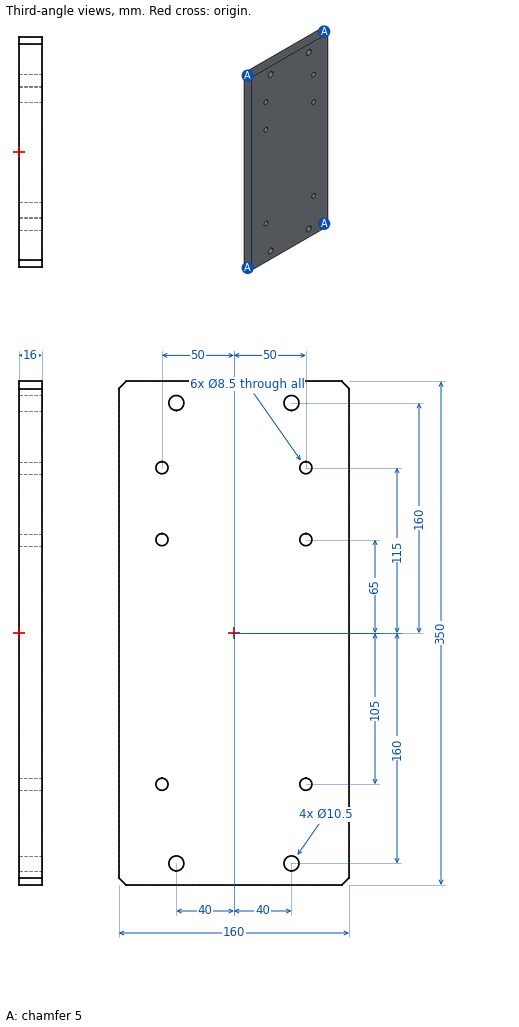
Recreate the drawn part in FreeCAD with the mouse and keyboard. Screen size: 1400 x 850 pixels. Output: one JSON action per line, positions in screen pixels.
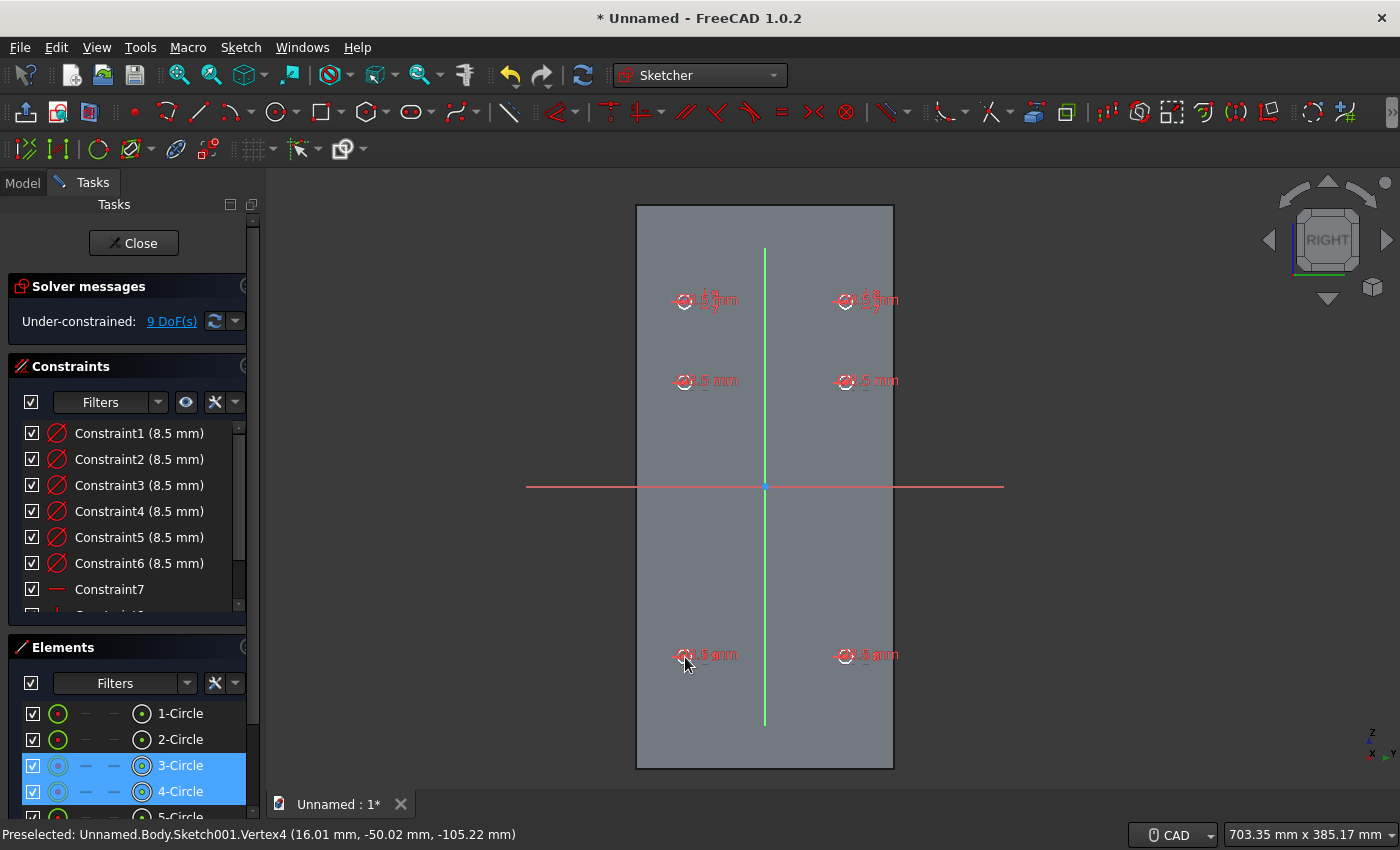
{"action": "left_click", "coordinate": [664, 112]}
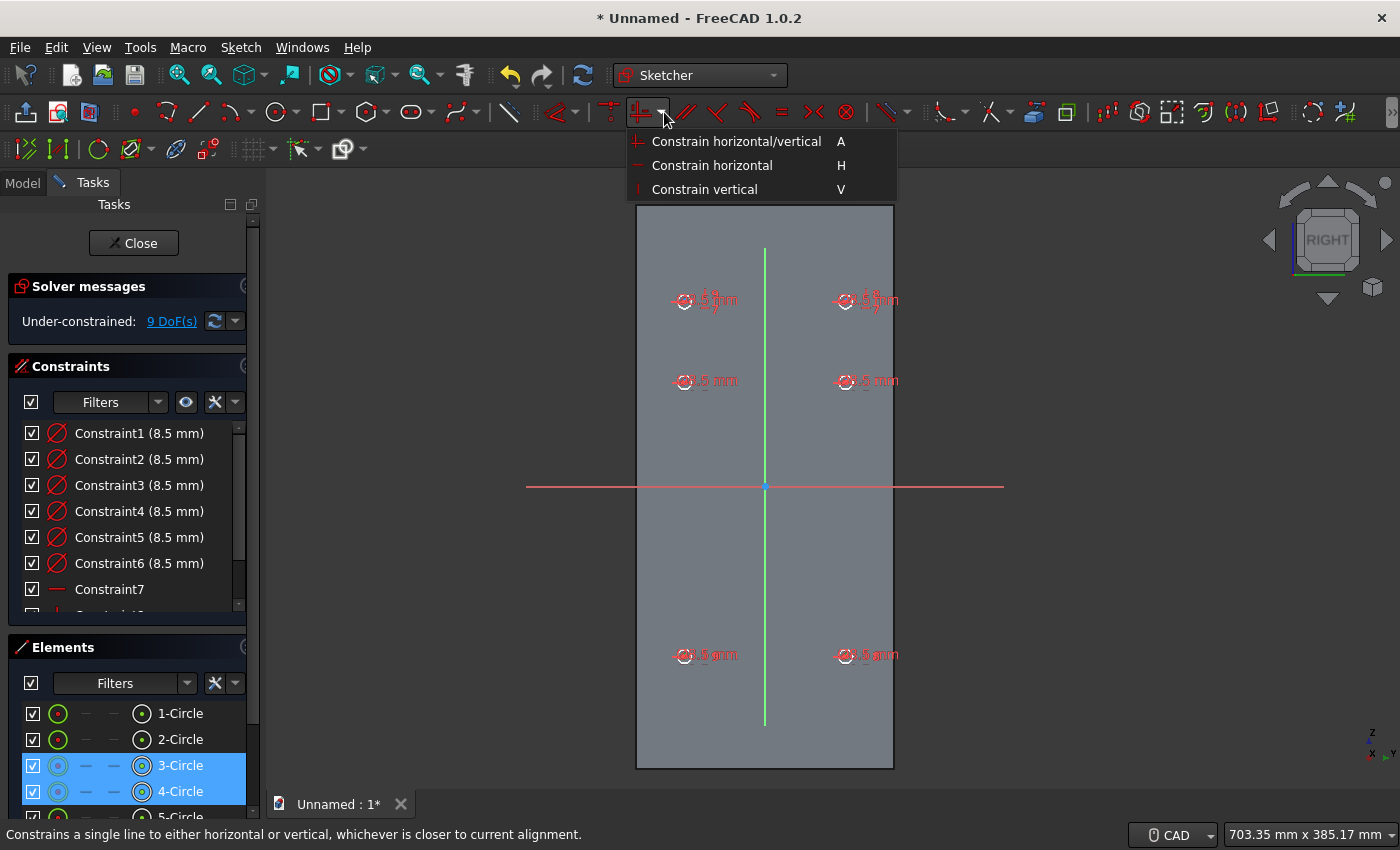
{"action": "left_click", "coordinate": [762, 165]}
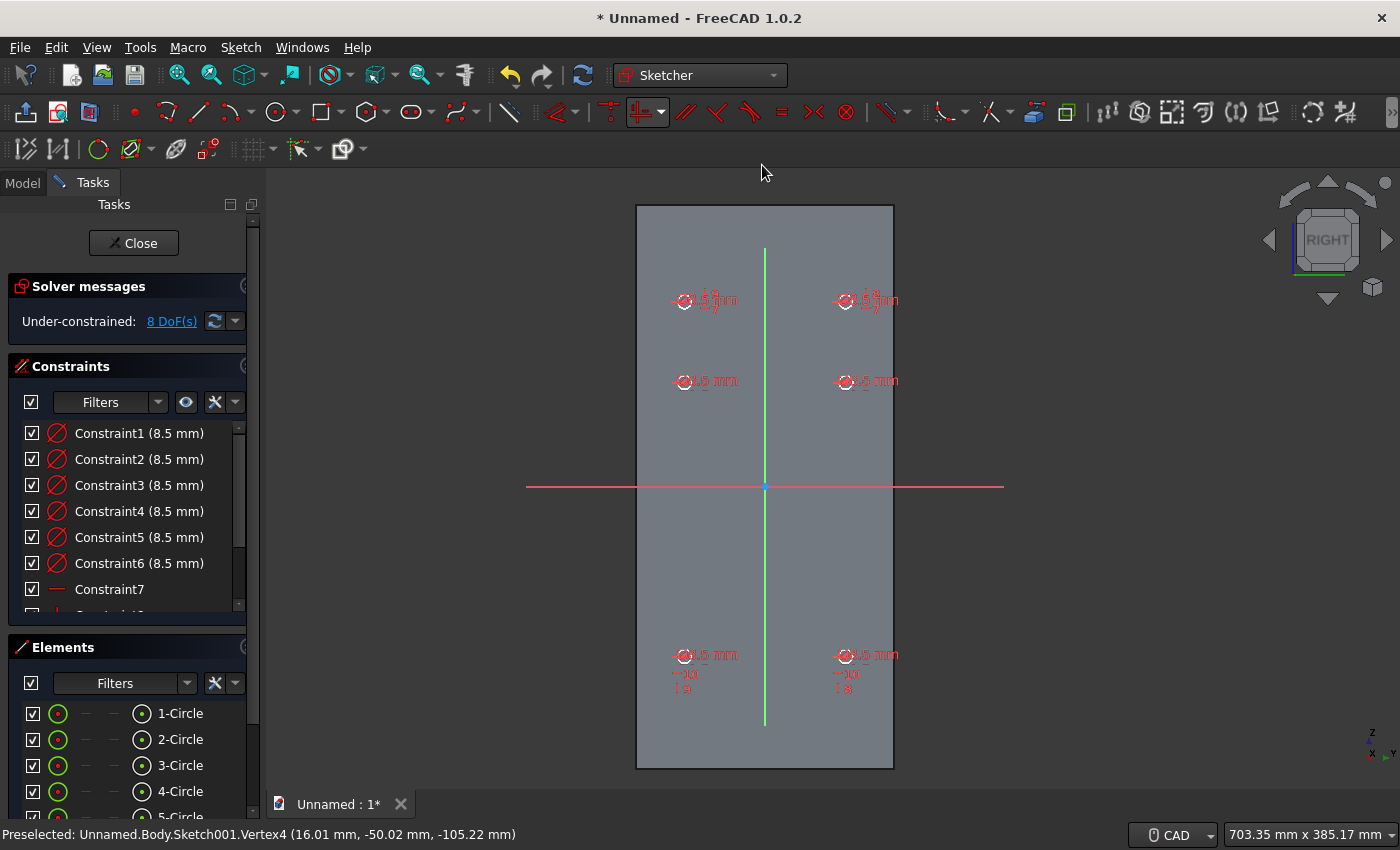
{"action": "left_click", "coordinate": [846, 302]}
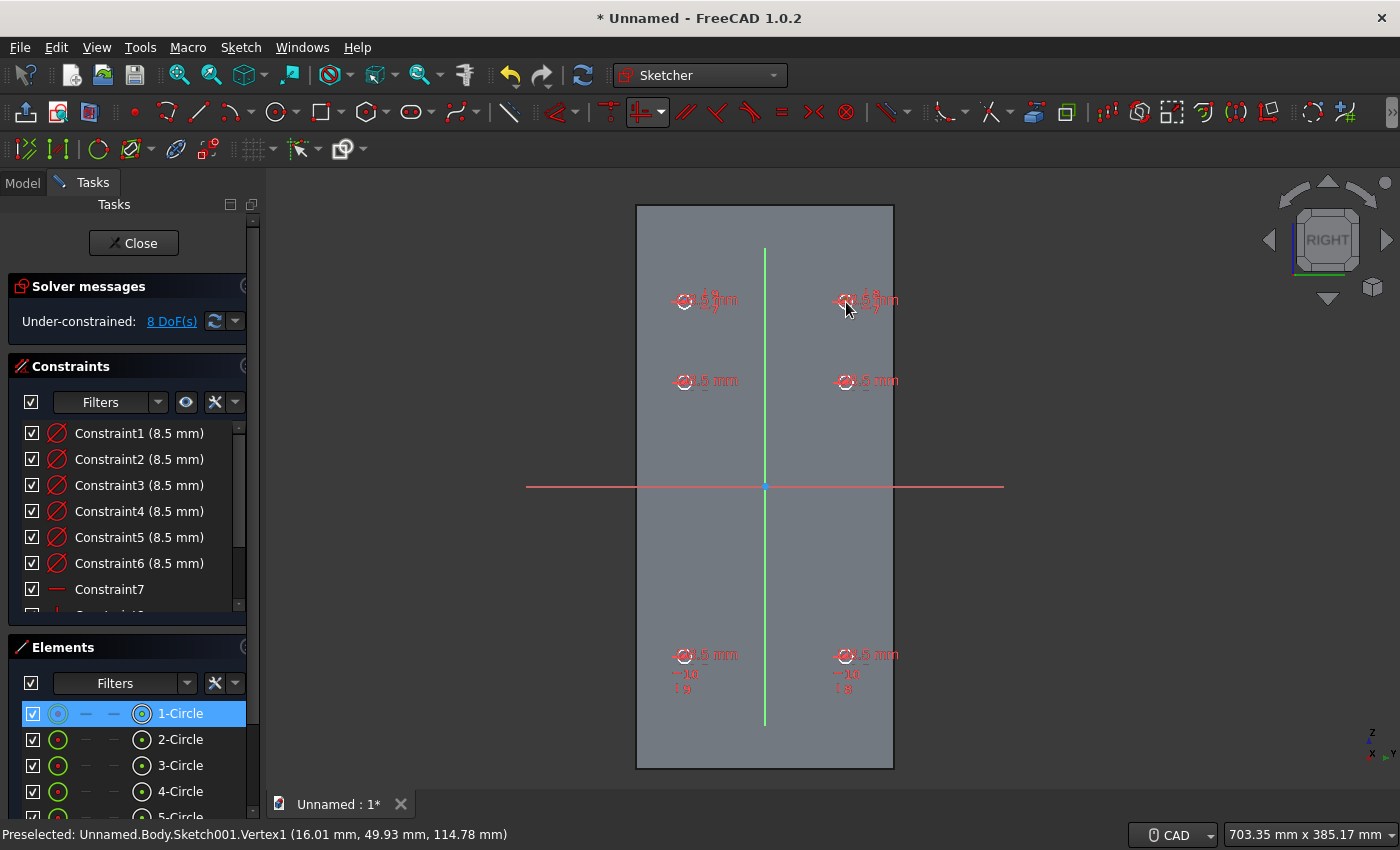
{"action": "left_click", "coordinate": [846, 383]}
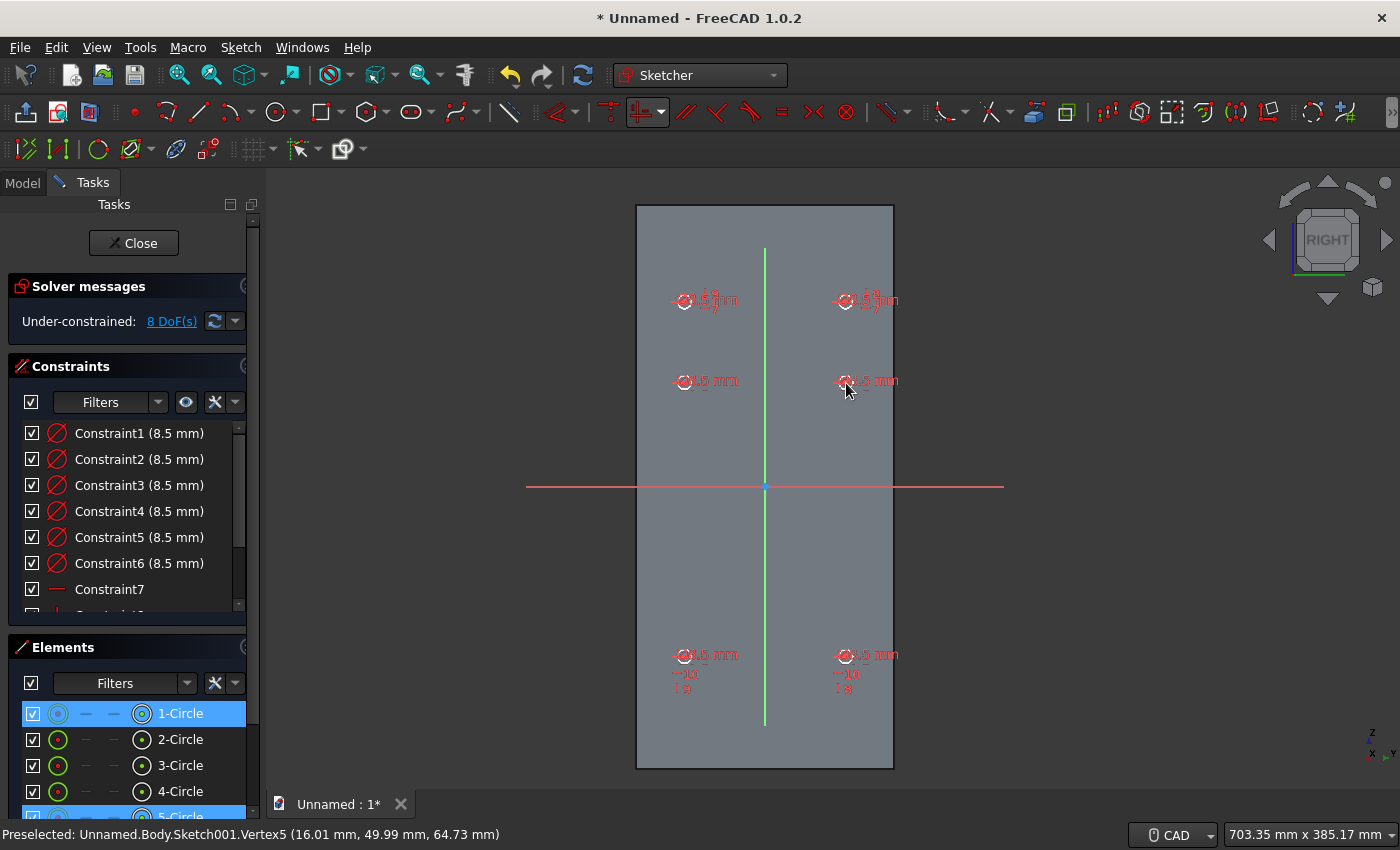
{"action": "key", "text": "v"}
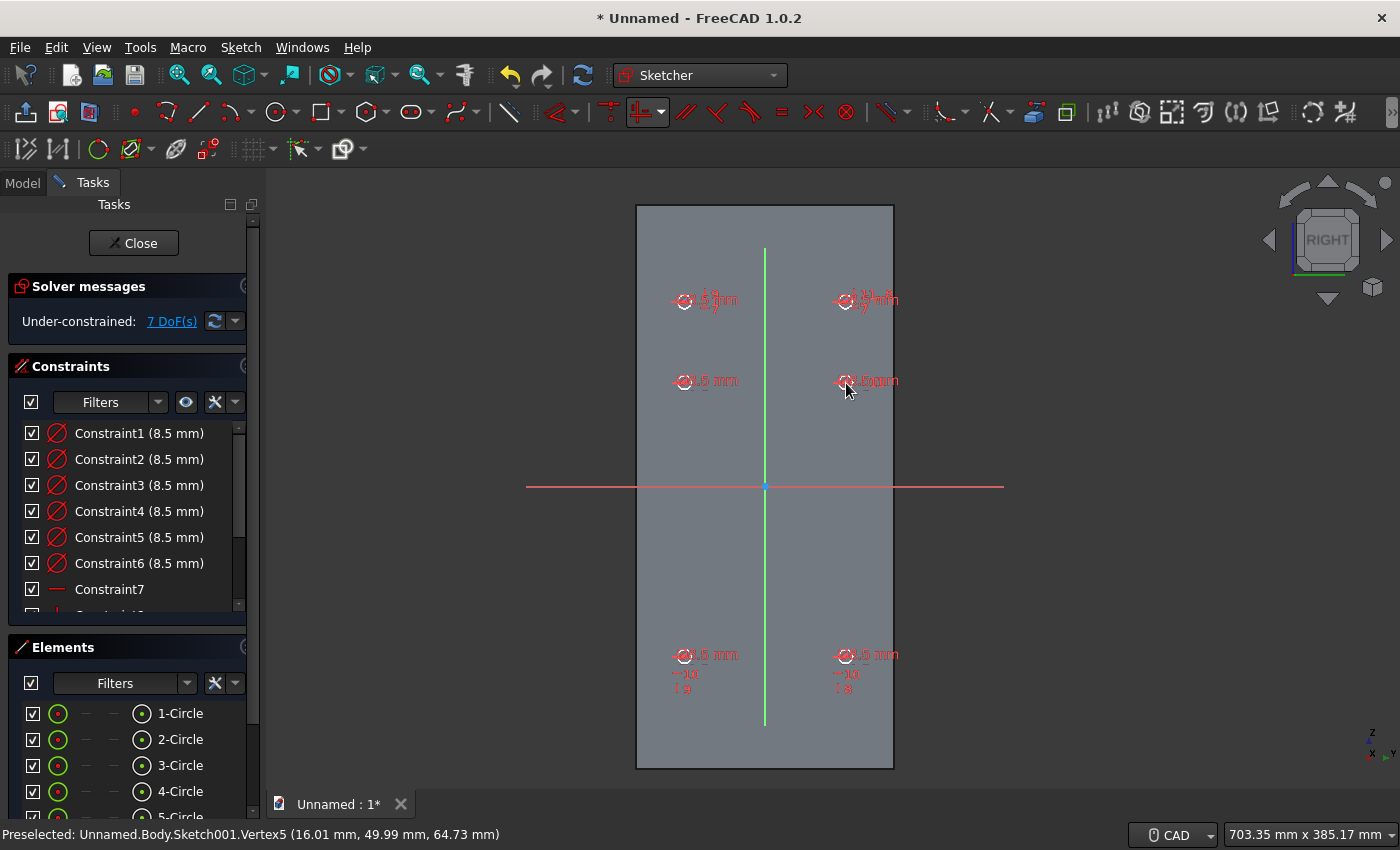
{"action": "left_click", "coordinate": [685, 302]}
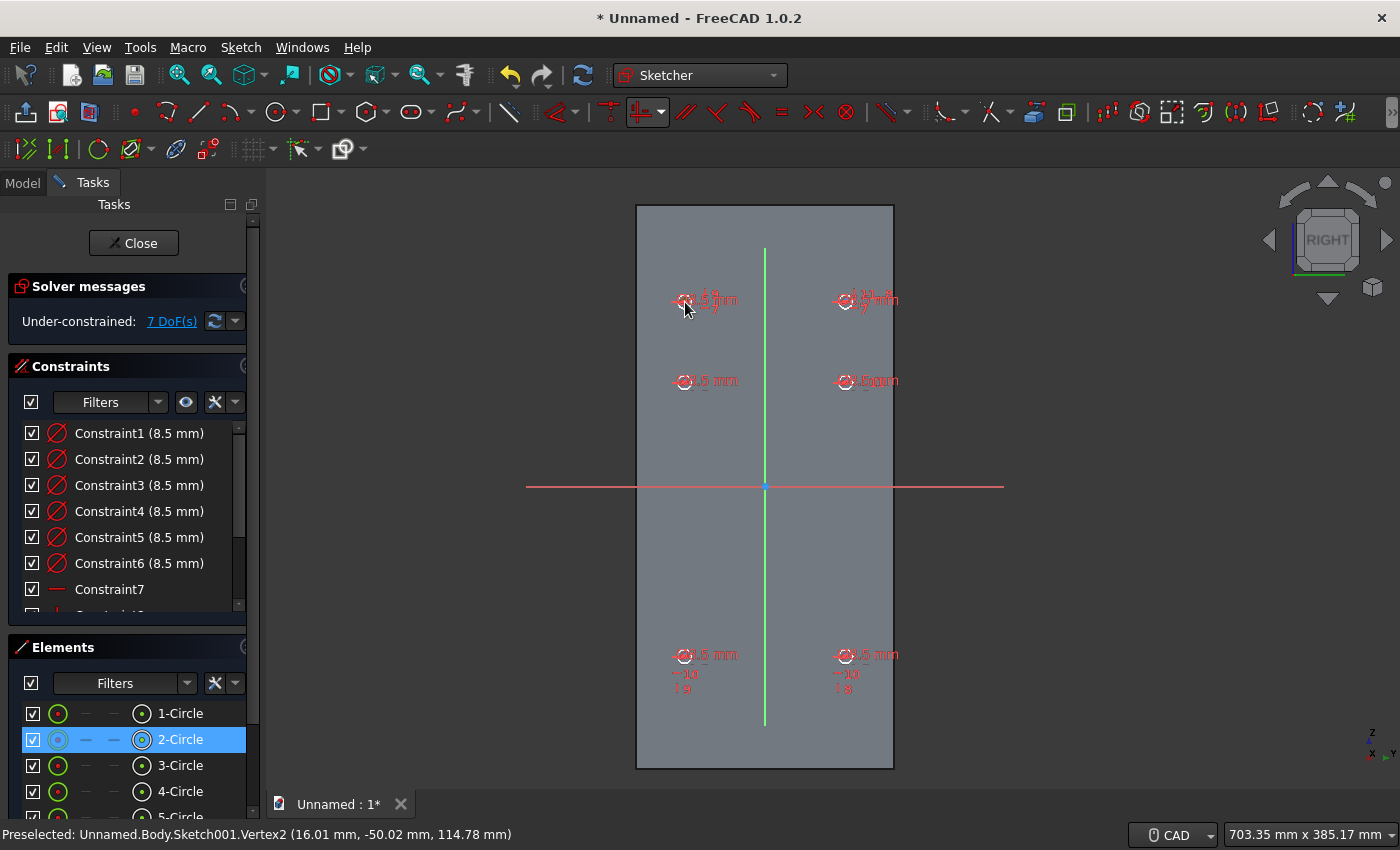
{"action": "left_click", "coordinate": [685, 383]}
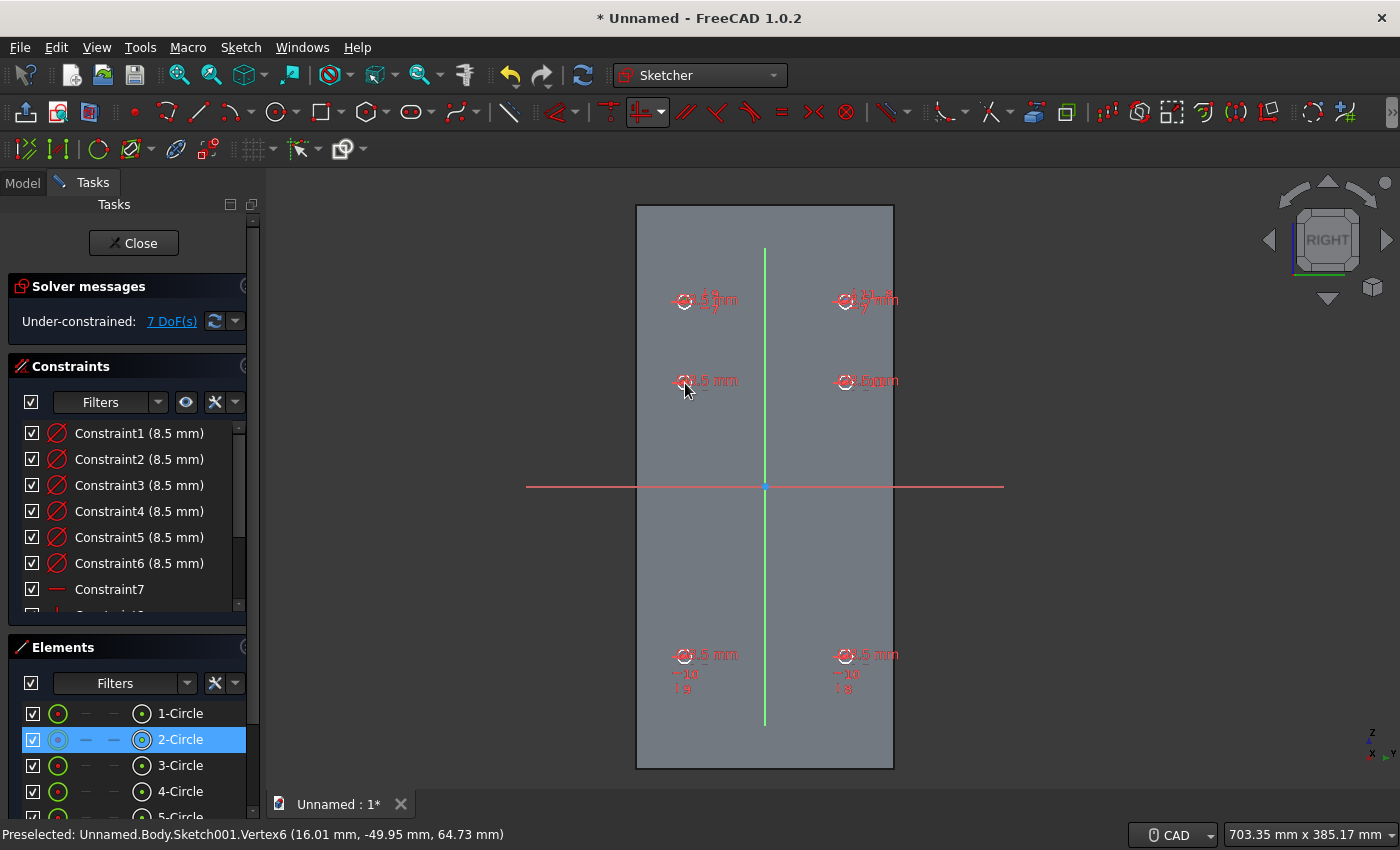
{"action": "key", "text": "v"}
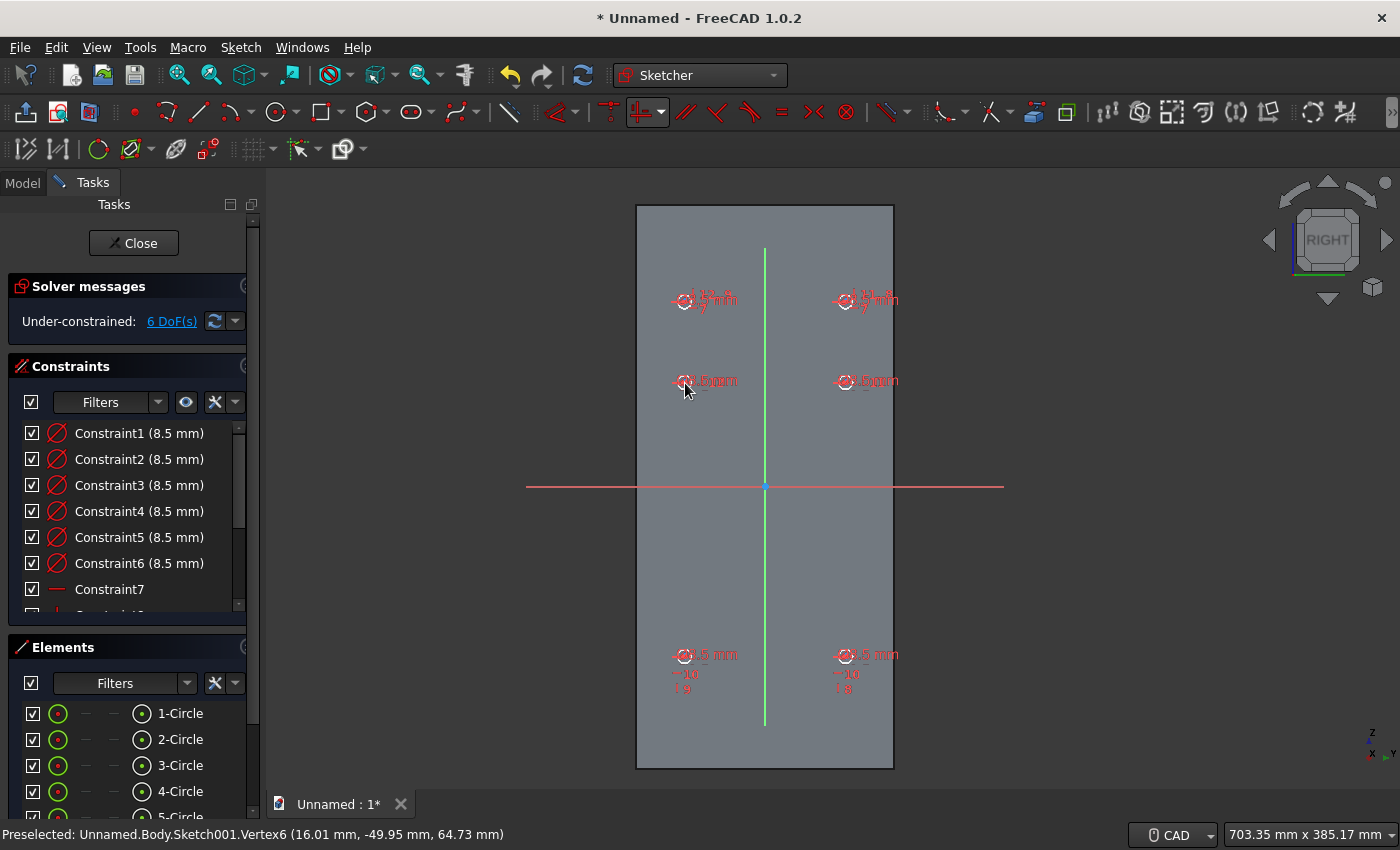
{"action": "left_click", "coordinate": [846, 383]}